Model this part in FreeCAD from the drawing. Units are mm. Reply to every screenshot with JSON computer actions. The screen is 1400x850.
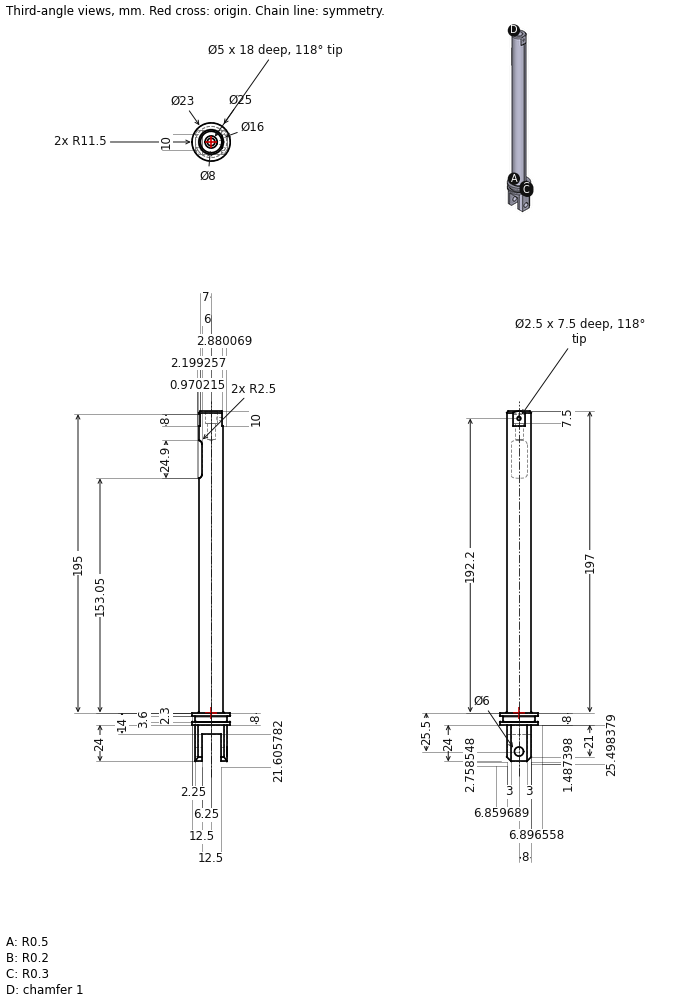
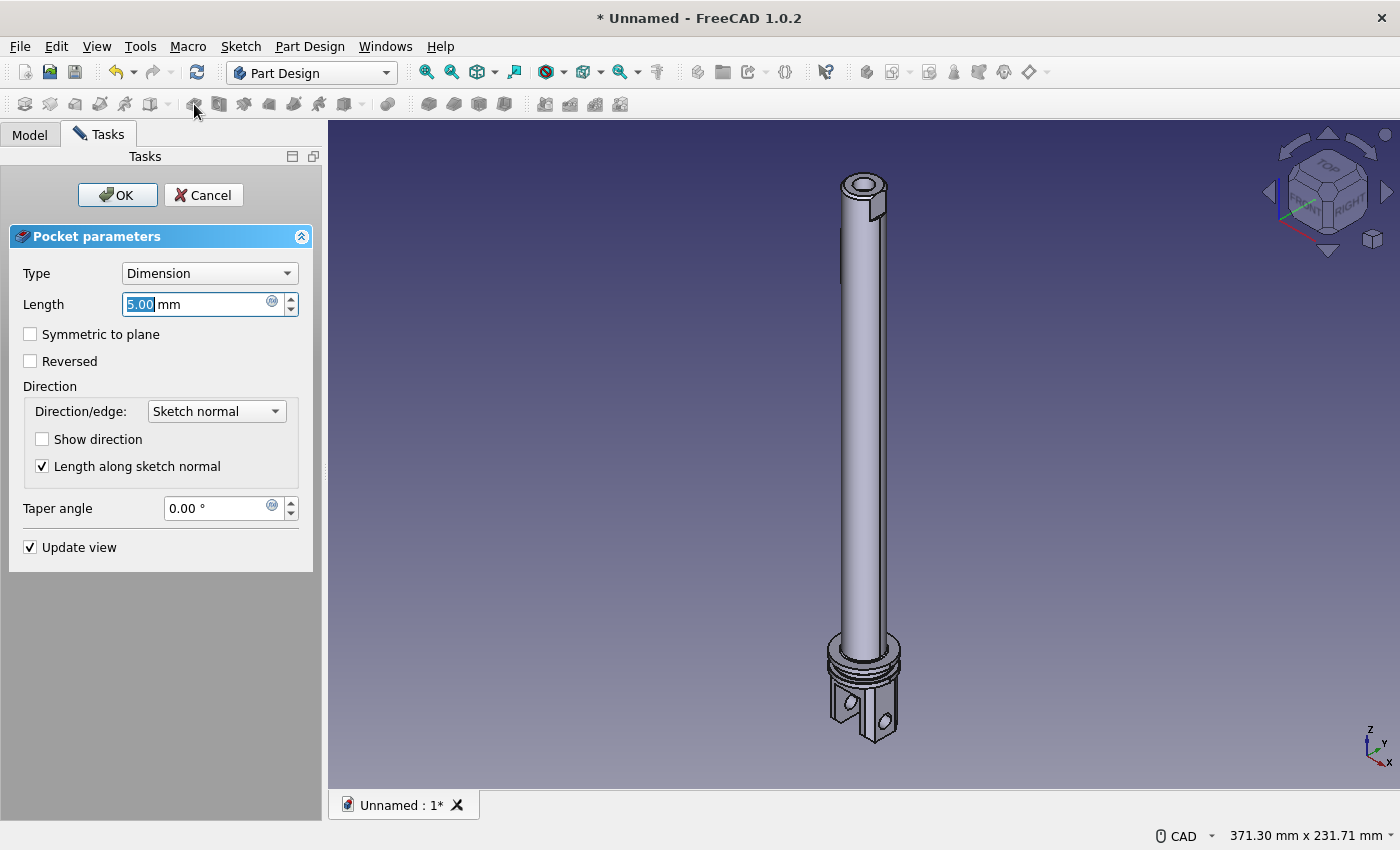
{"action": "type", "text": "7.5"}
{"action": "key", "text": "Tab"}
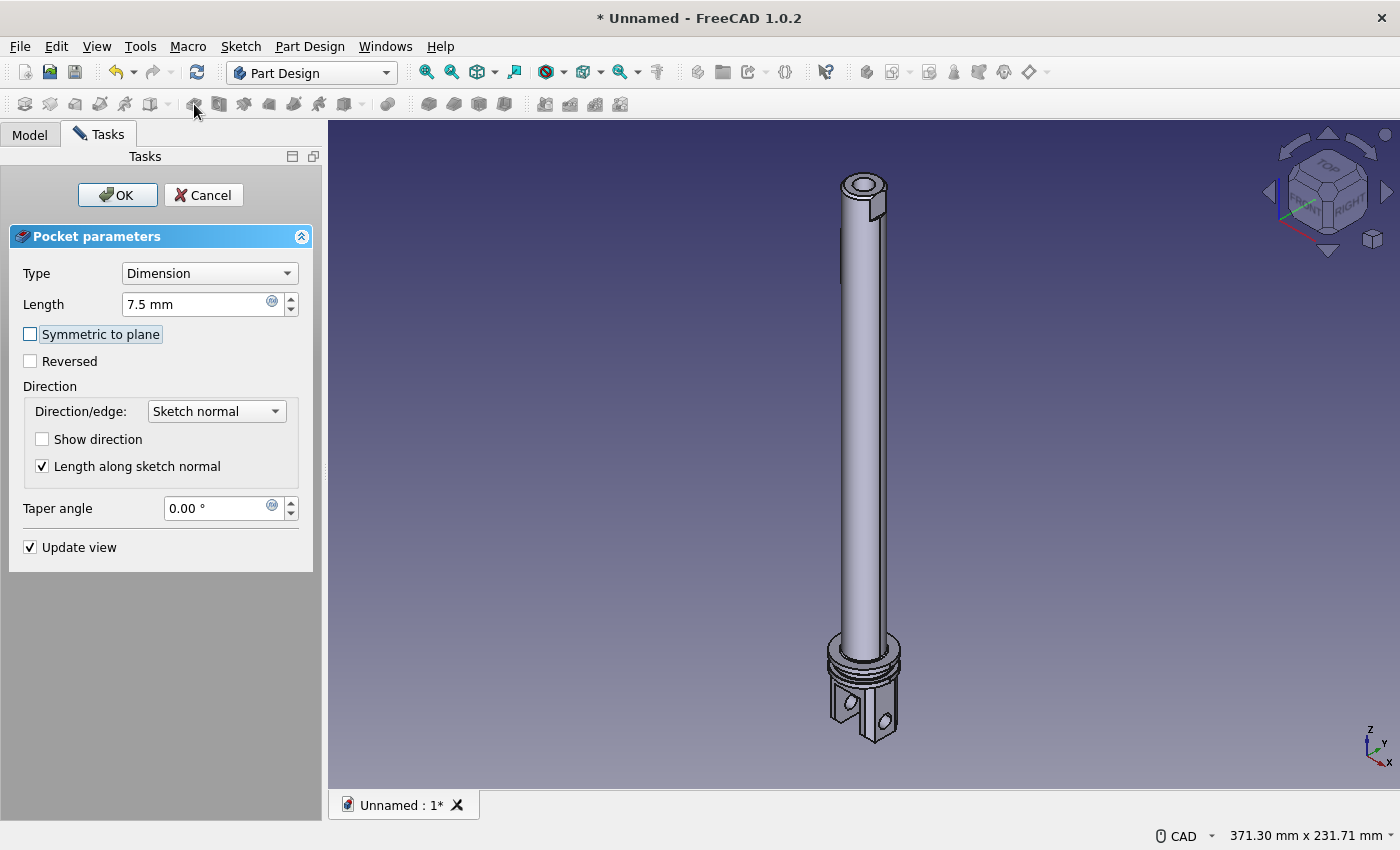
{"action": "left_click", "coordinate": [118, 195]}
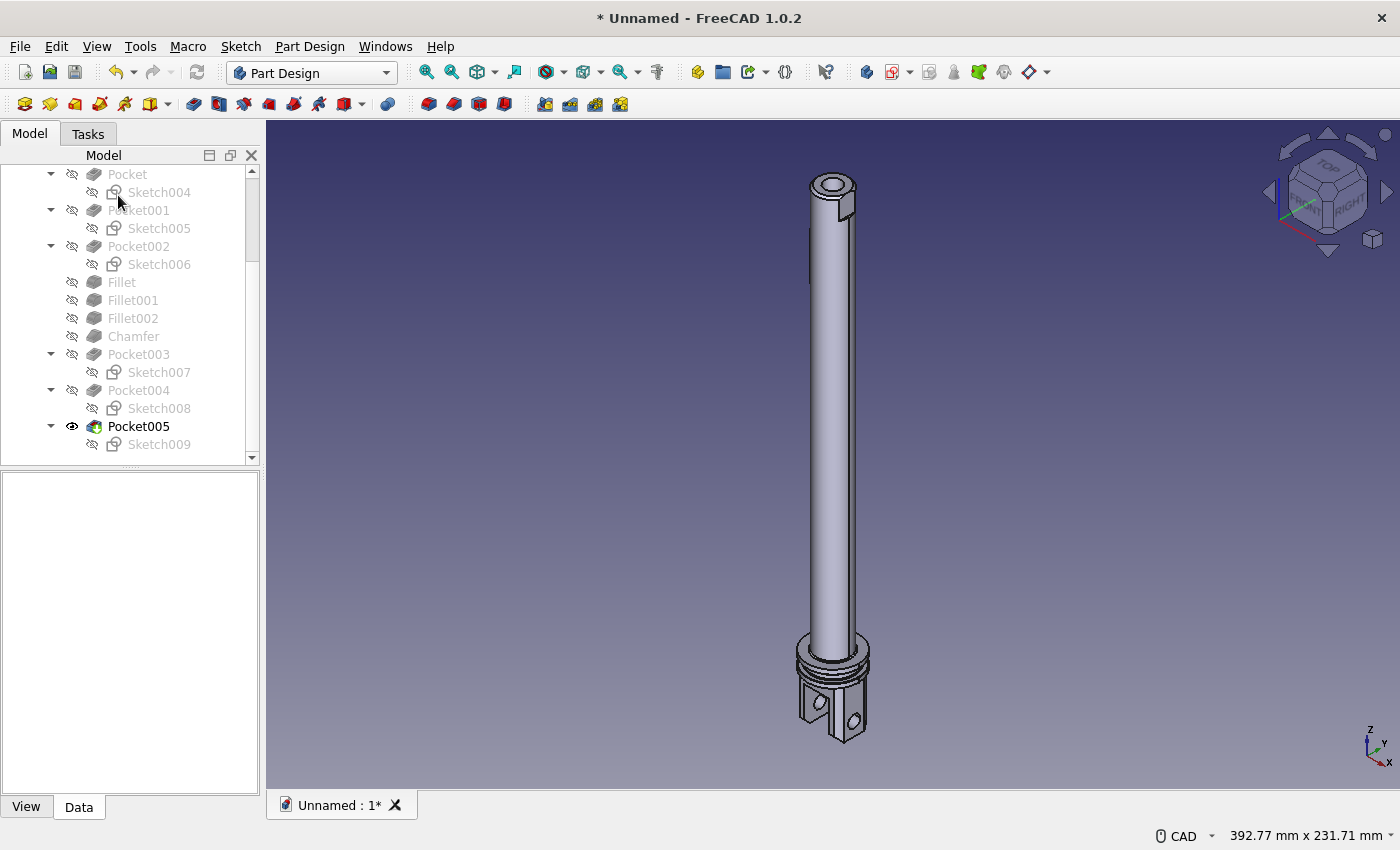
{"action": "scroll", "coordinate": [817, 184], "scroll_direction": "up", "scroll_amount": 6}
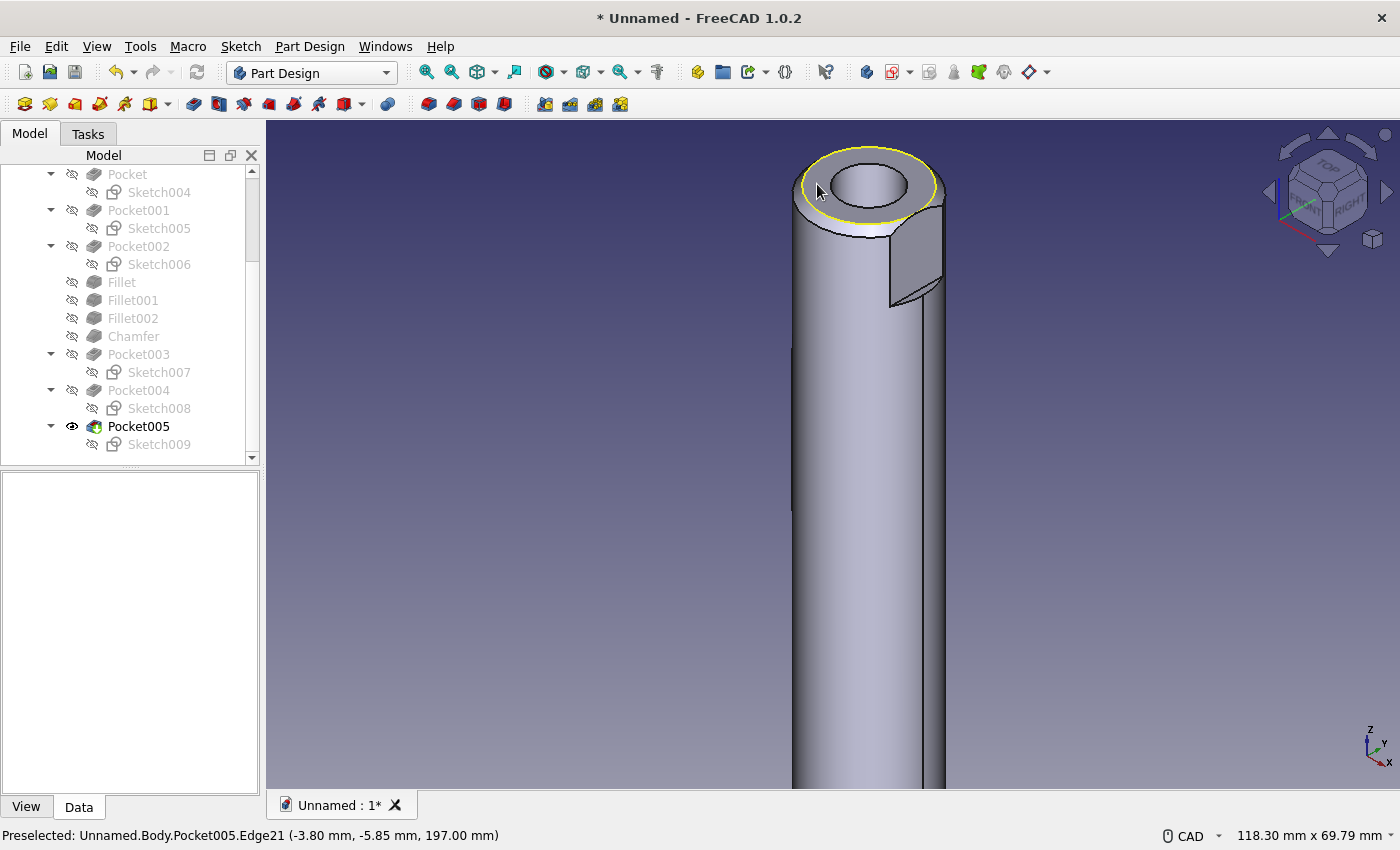
{"action": "left_click", "coordinate": [815, 185]}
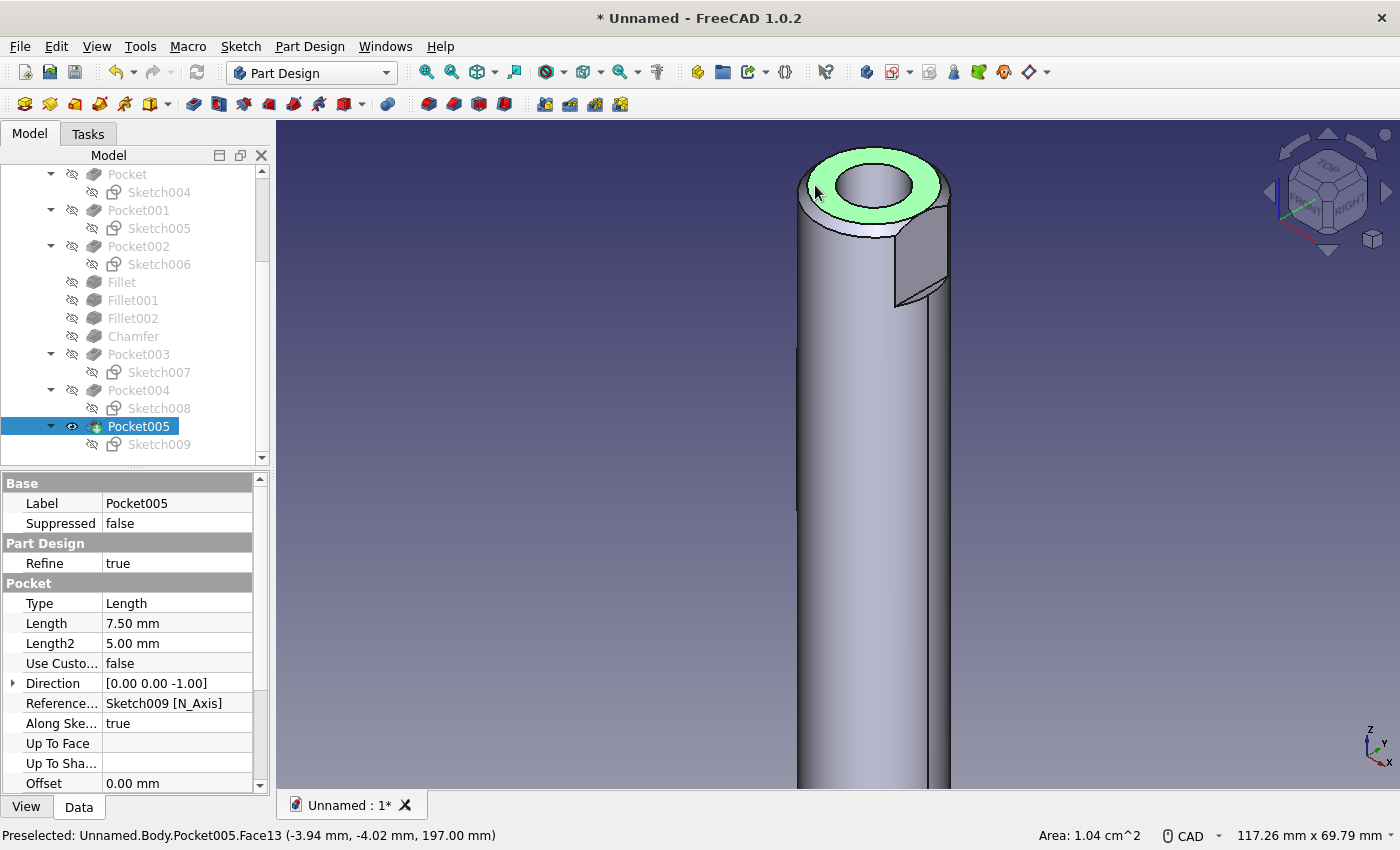
{"action": "left_click", "coordinate": [892, 72]}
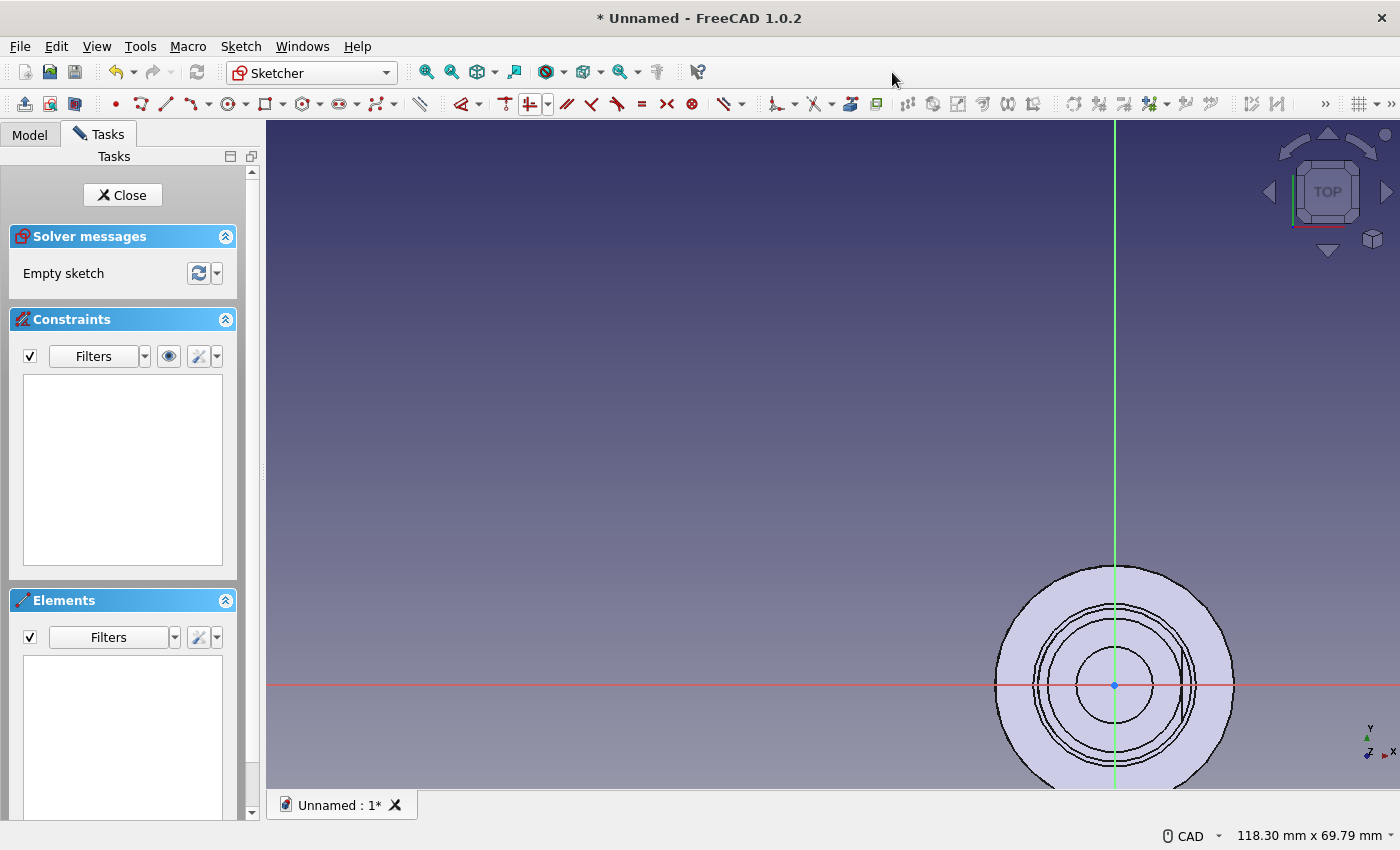
{"action": "scroll", "coordinate": [1158, 714], "scroll_direction": "up", "scroll_amount": 11}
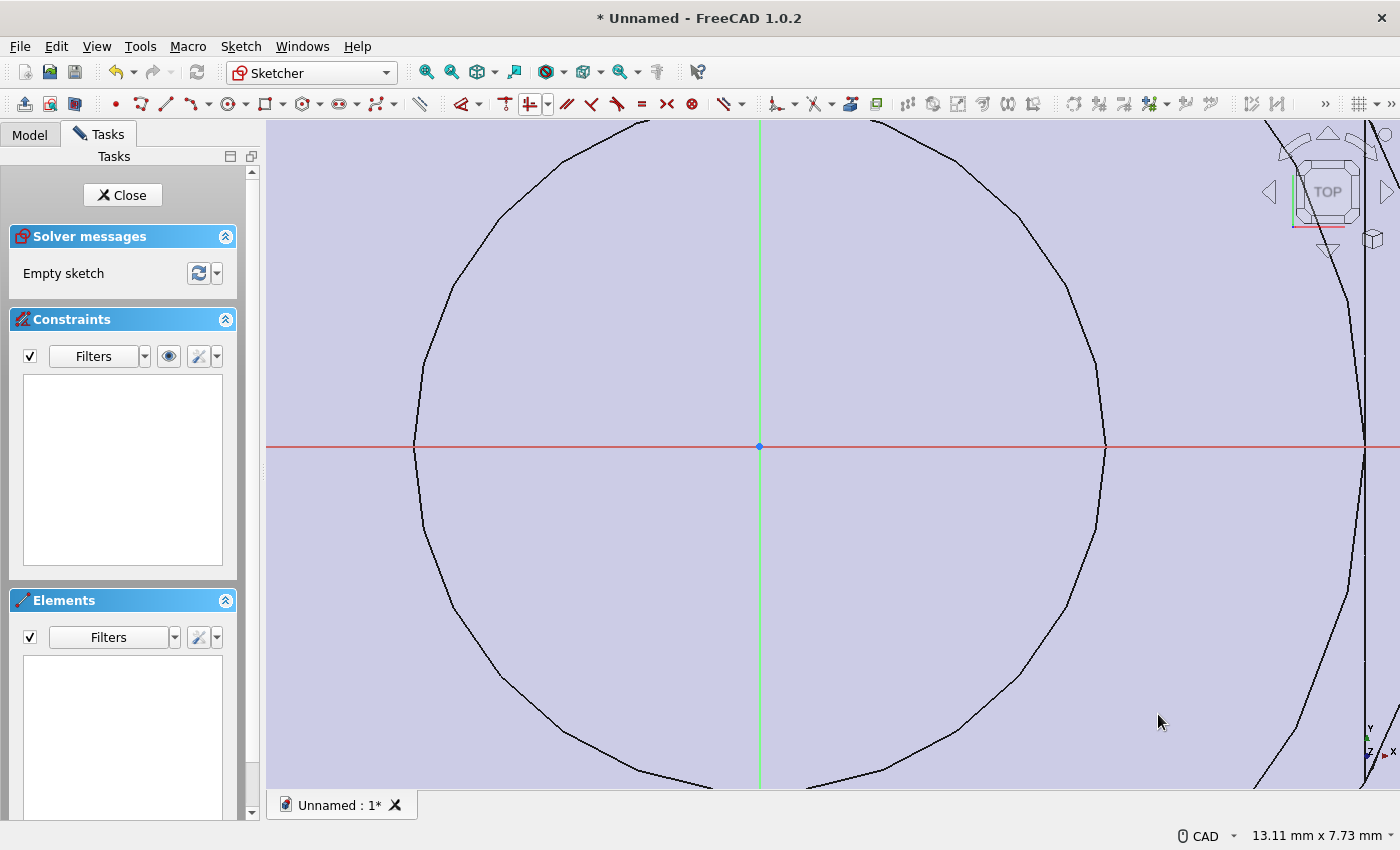
{"action": "left_click", "coordinate": [228, 104]}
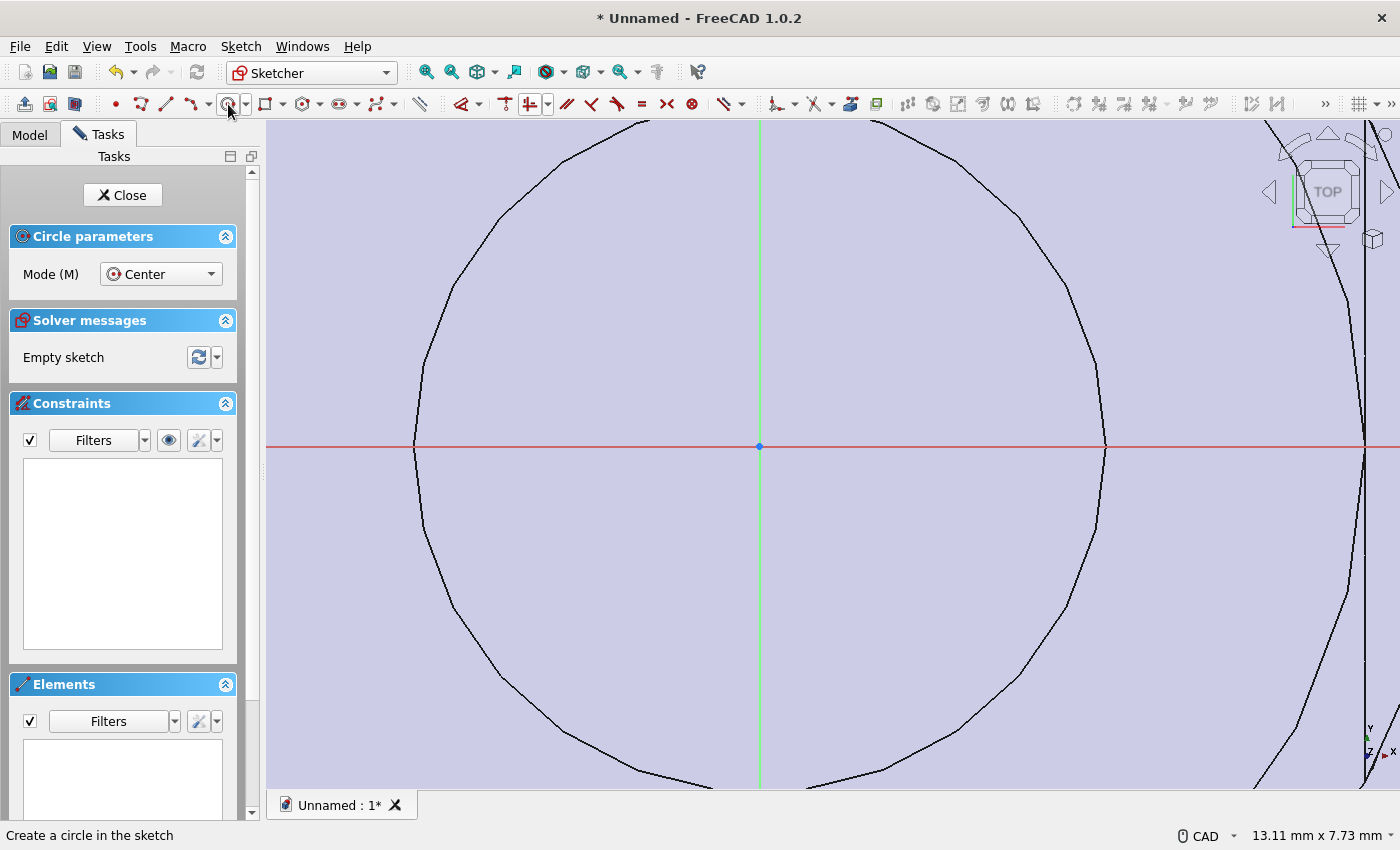
{"action": "left_click", "coordinate": [760, 447]}
{"action": "mouse_move", "coordinate": [913, 294]}